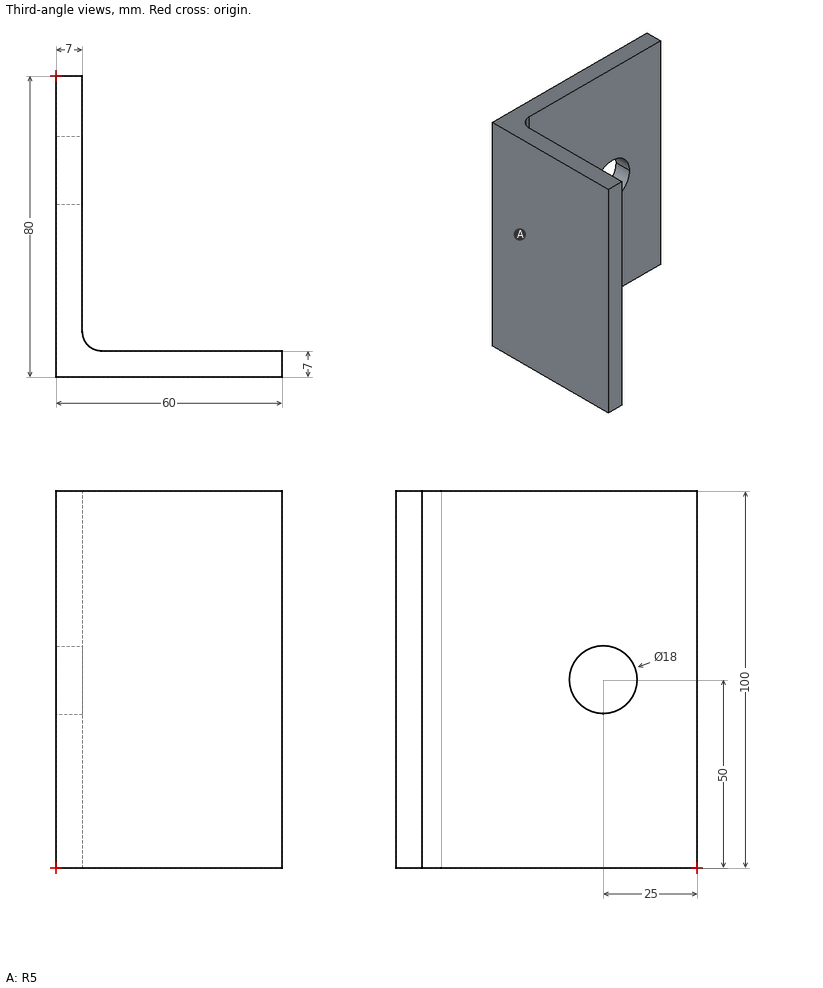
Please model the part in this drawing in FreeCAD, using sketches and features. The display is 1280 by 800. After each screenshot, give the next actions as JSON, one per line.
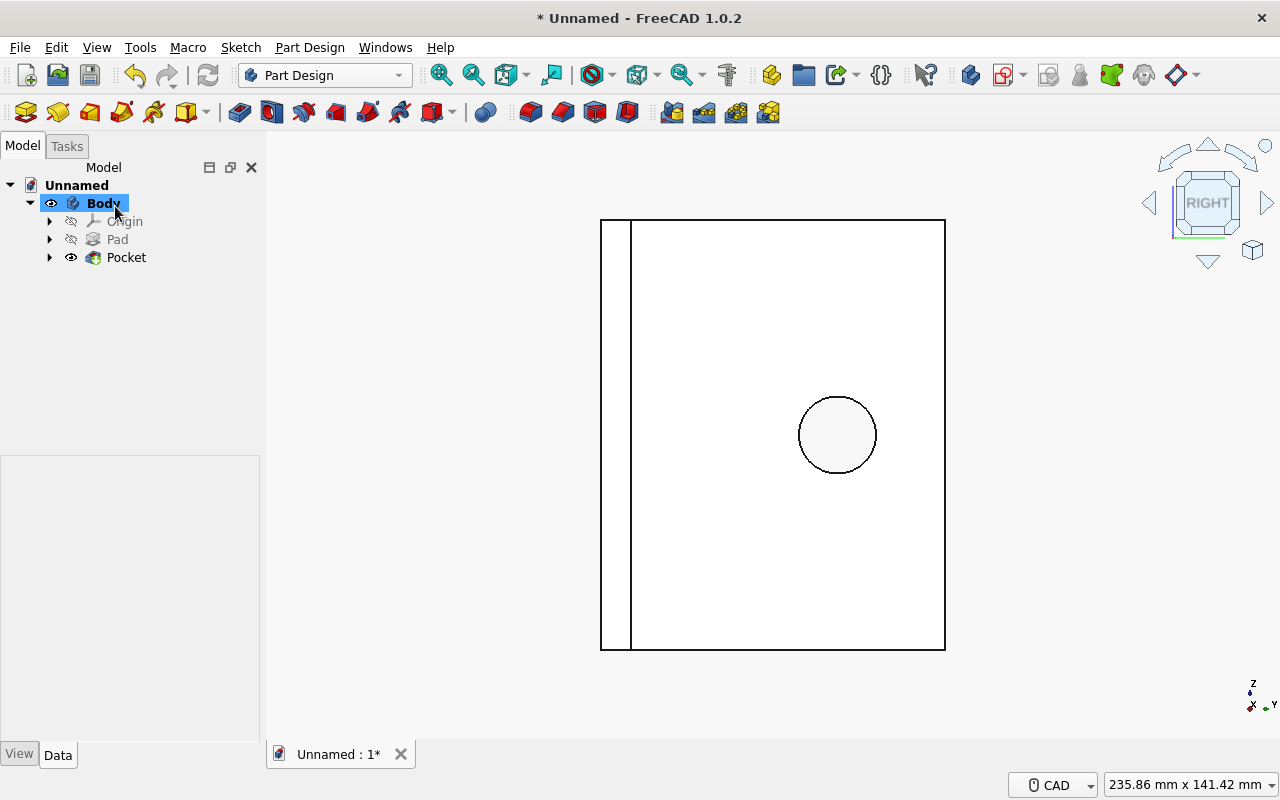
{"action": "key", "text": "5"}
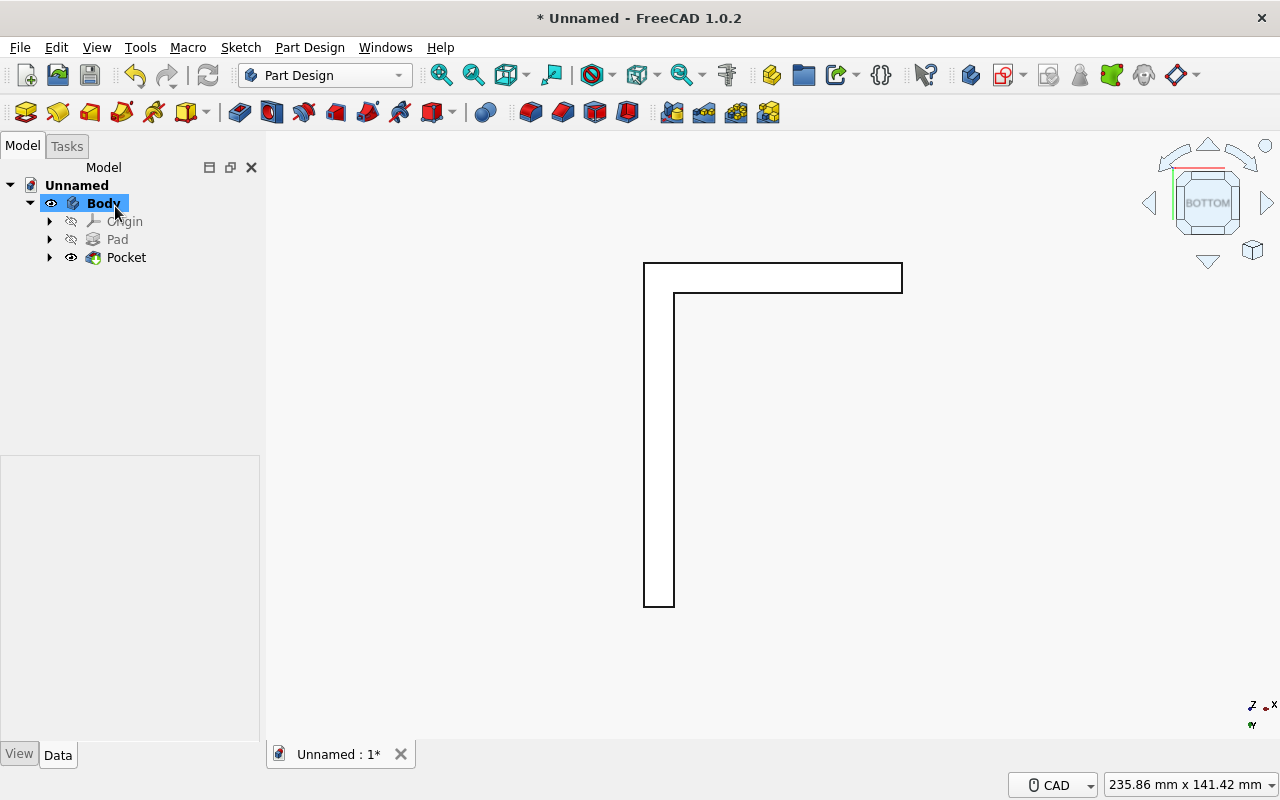
{"action": "key", "text": "4"}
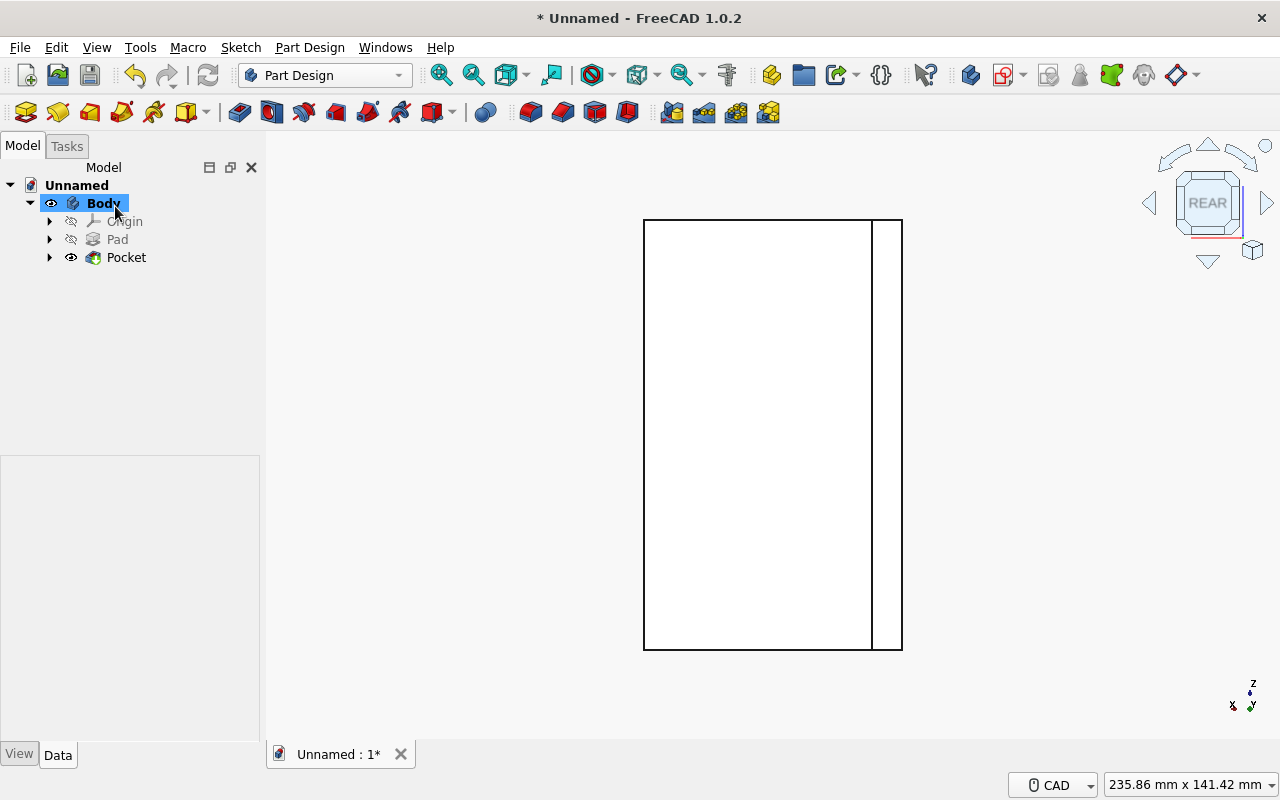
{"action": "key", "text": "6"}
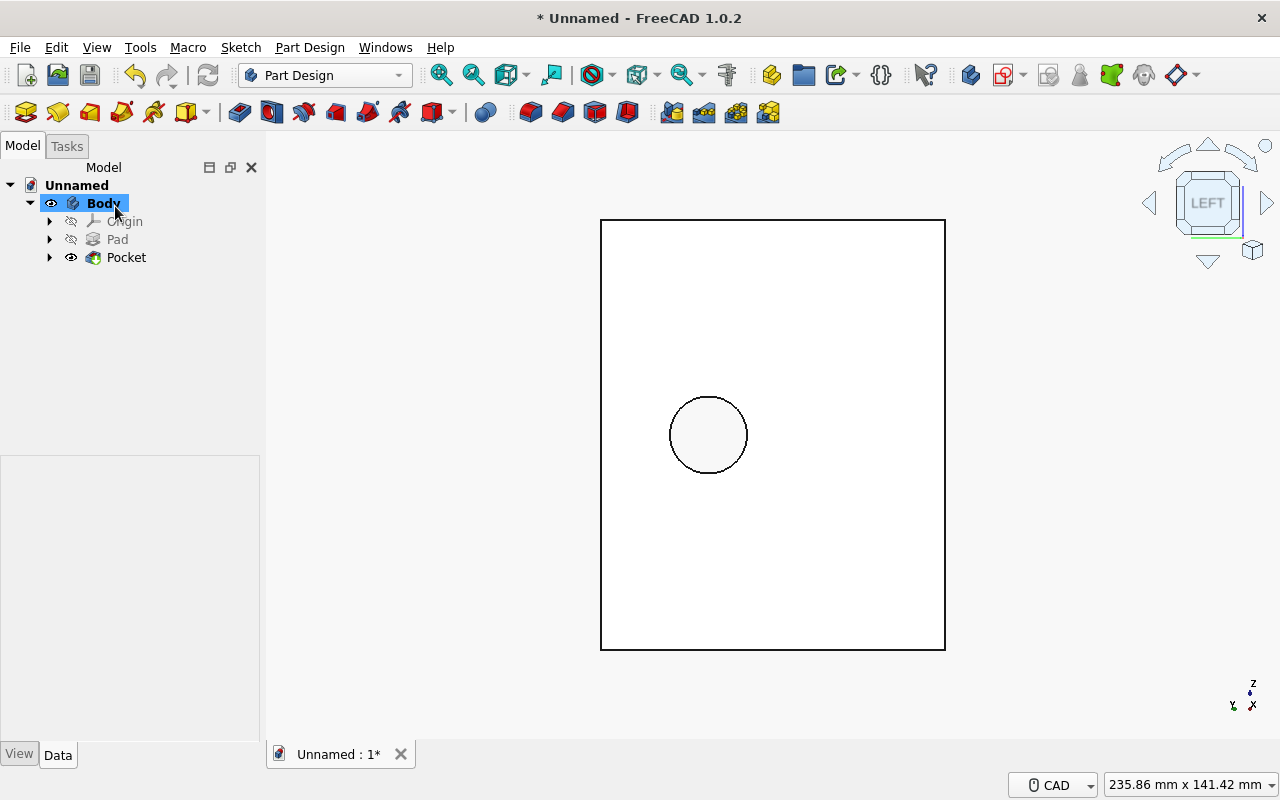
{"action": "key", "text": "v 3"}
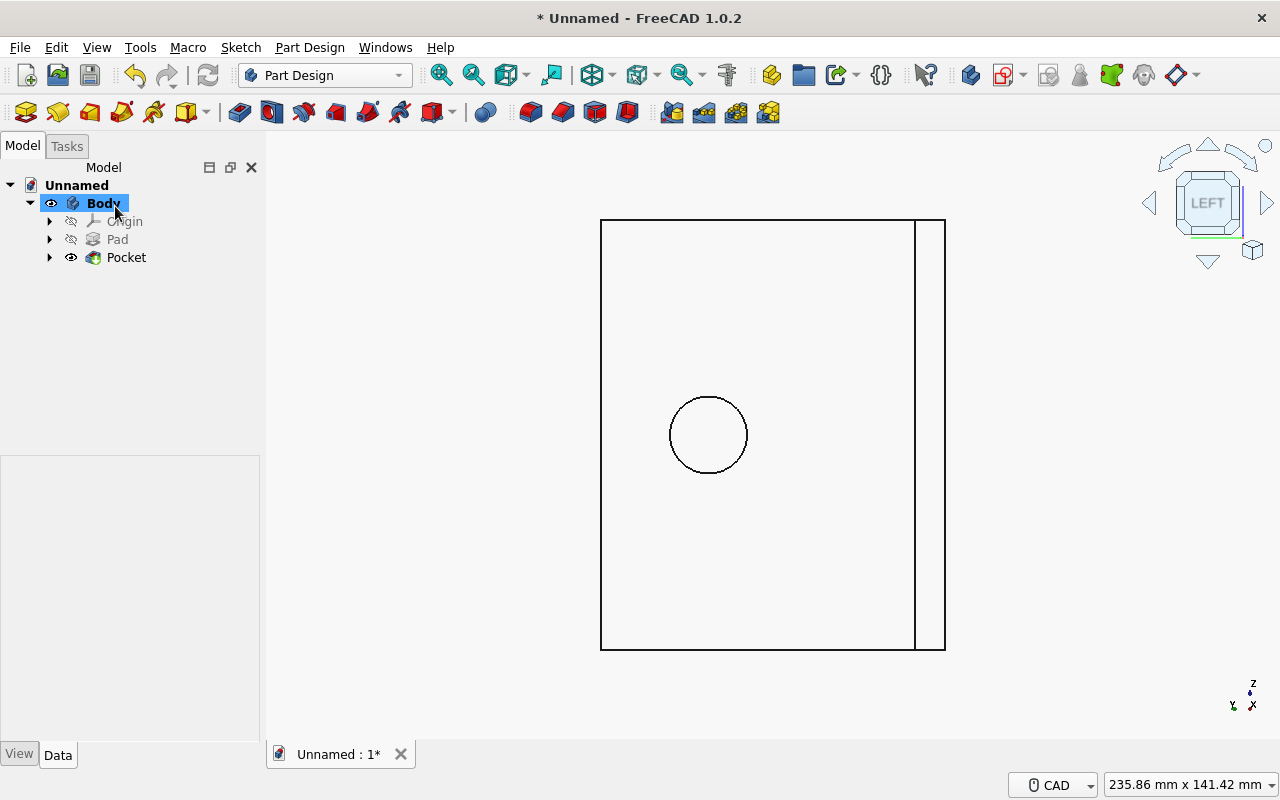
{"action": "key", "text": "0"}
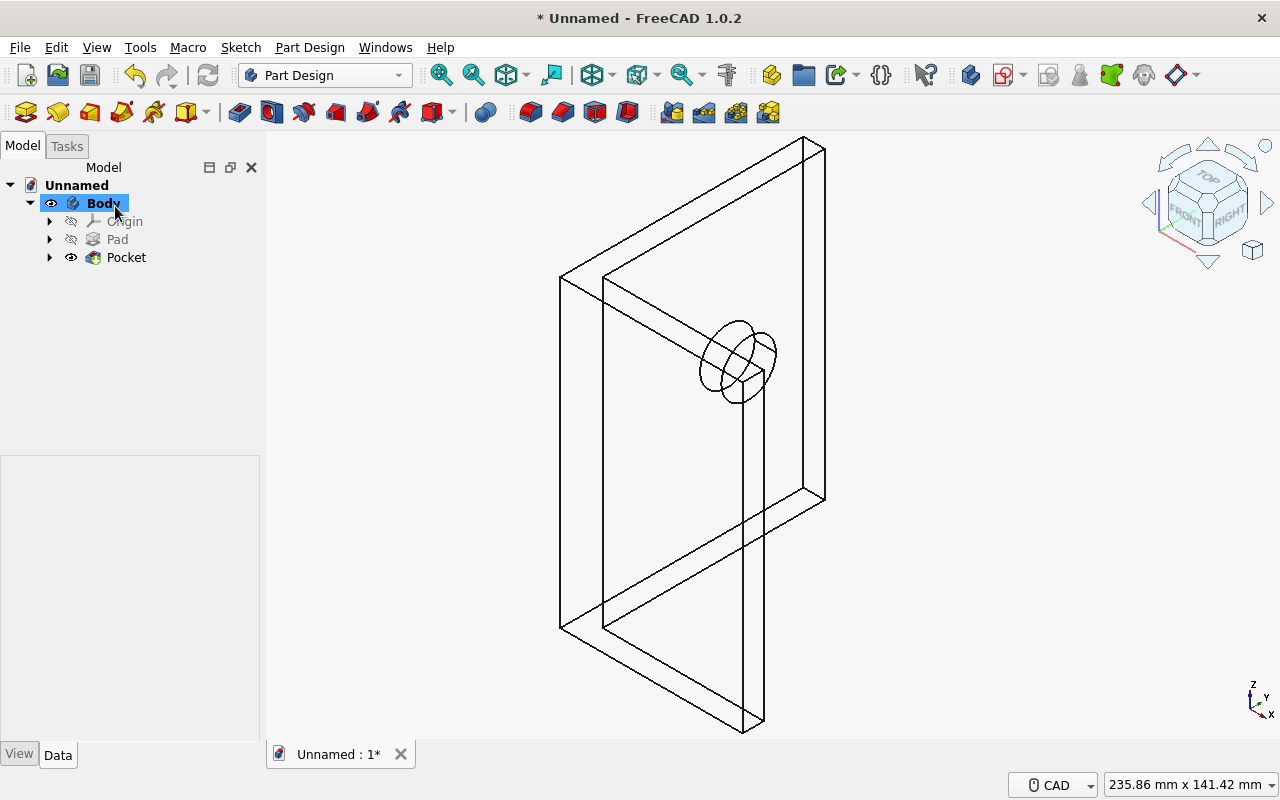
{"action": "left_click", "coordinate": [603, 452]}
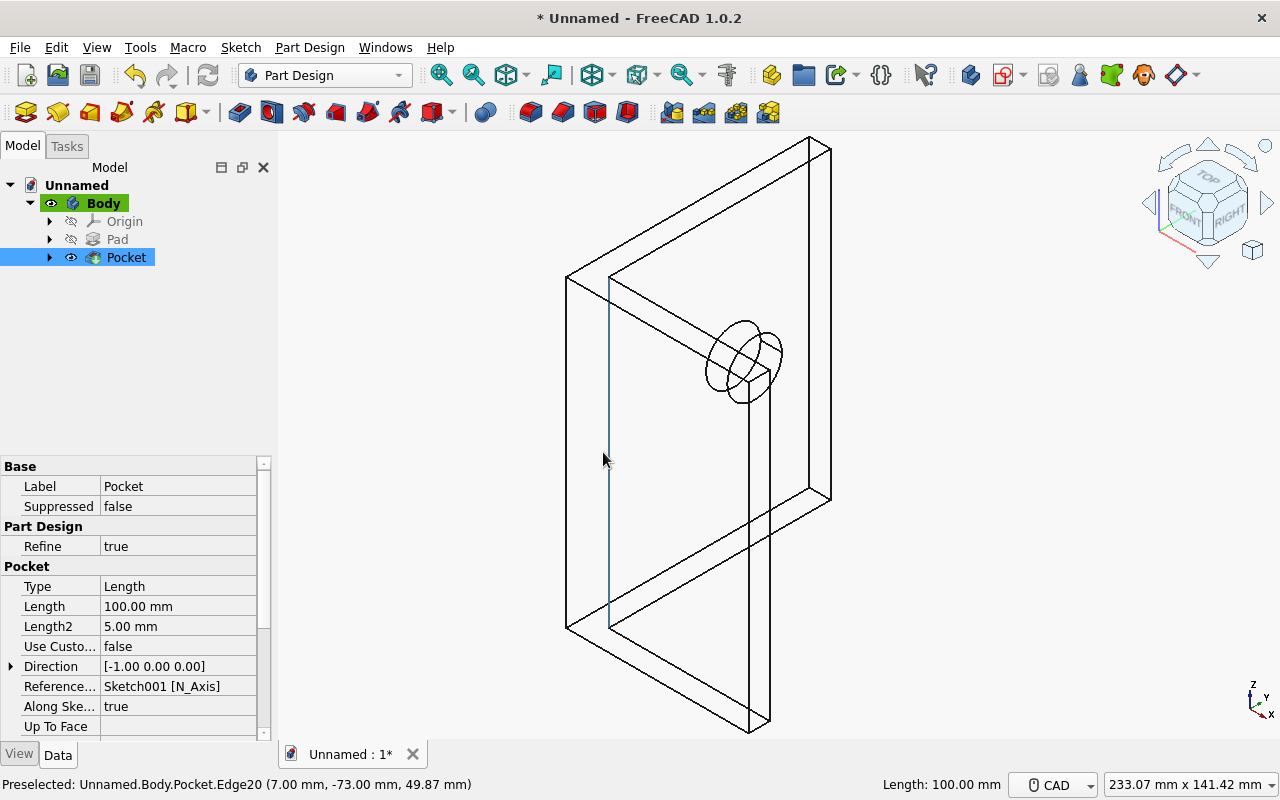
{"action": "key", "text": "v 1"}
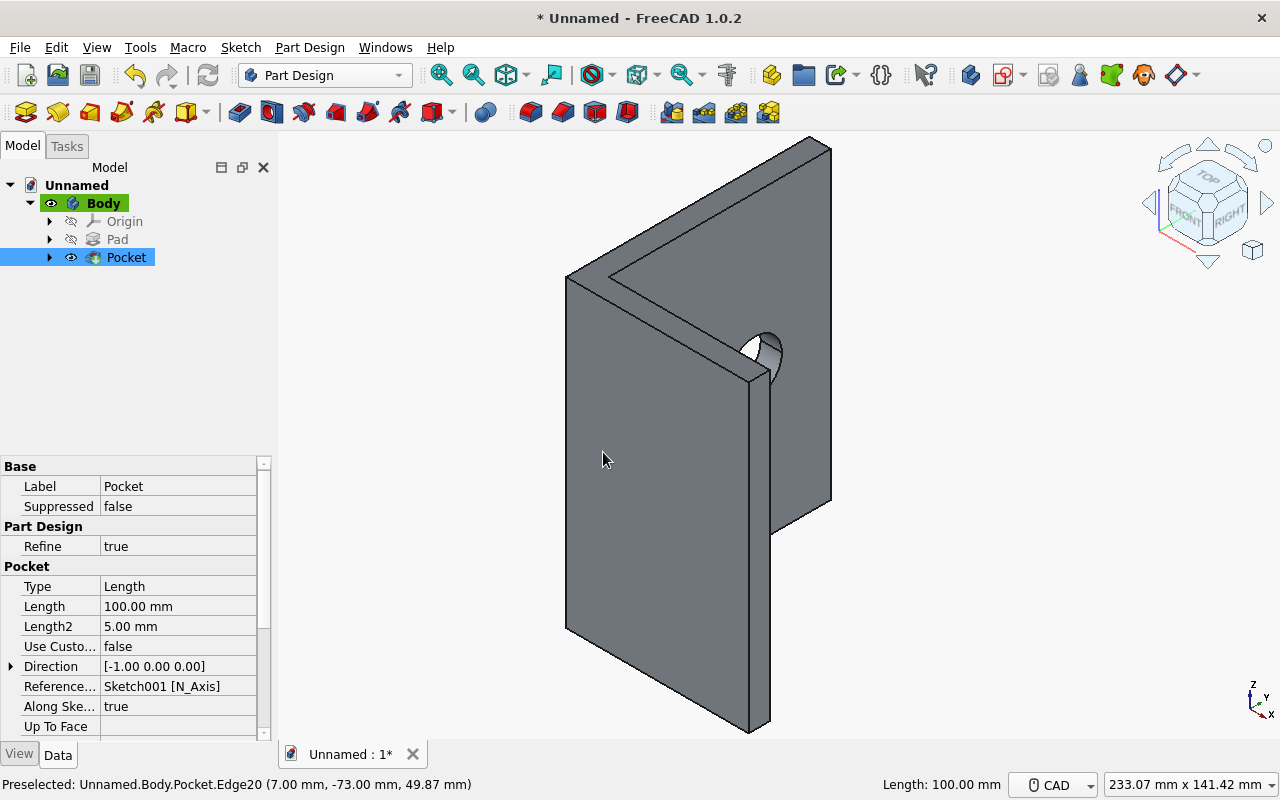
{"action": "left_click", "coordinate": [532, 112]}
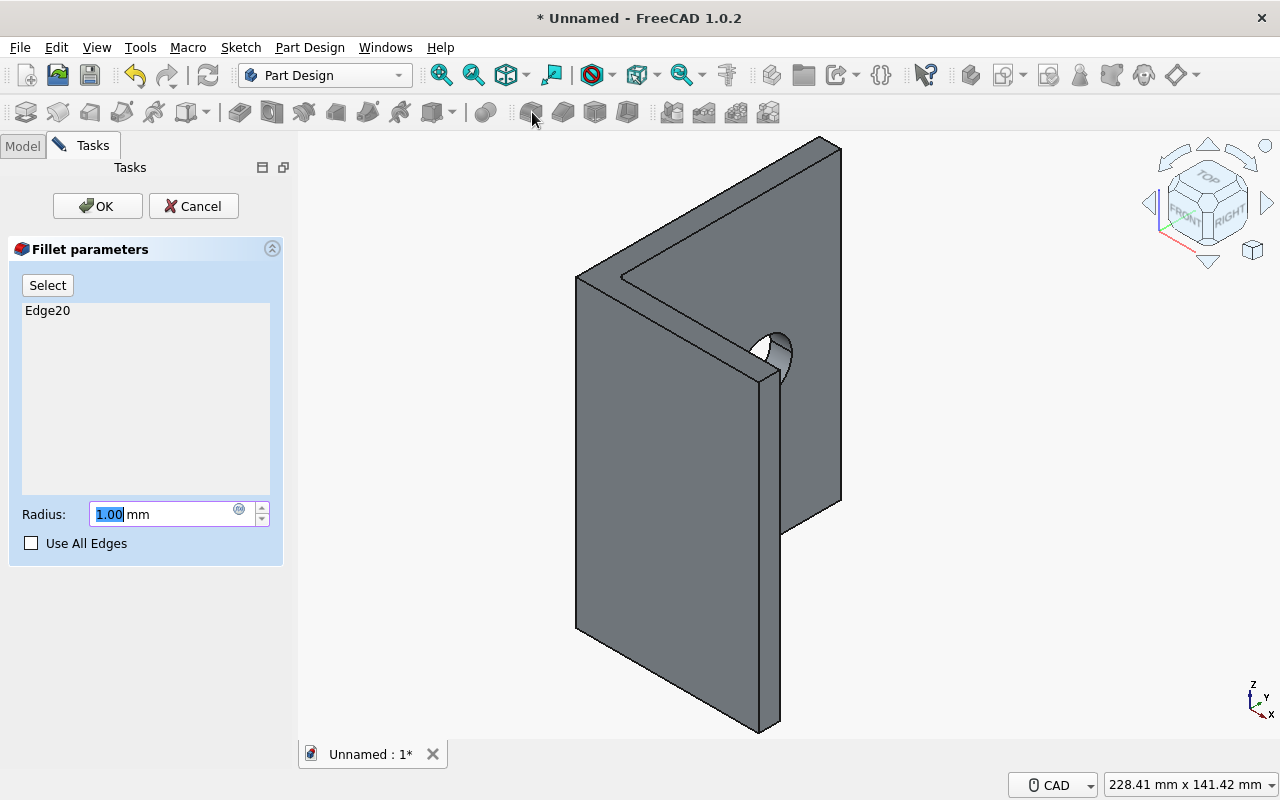
{"action": "type", "text": "5"}
{"action": "key", "text": "Tab"}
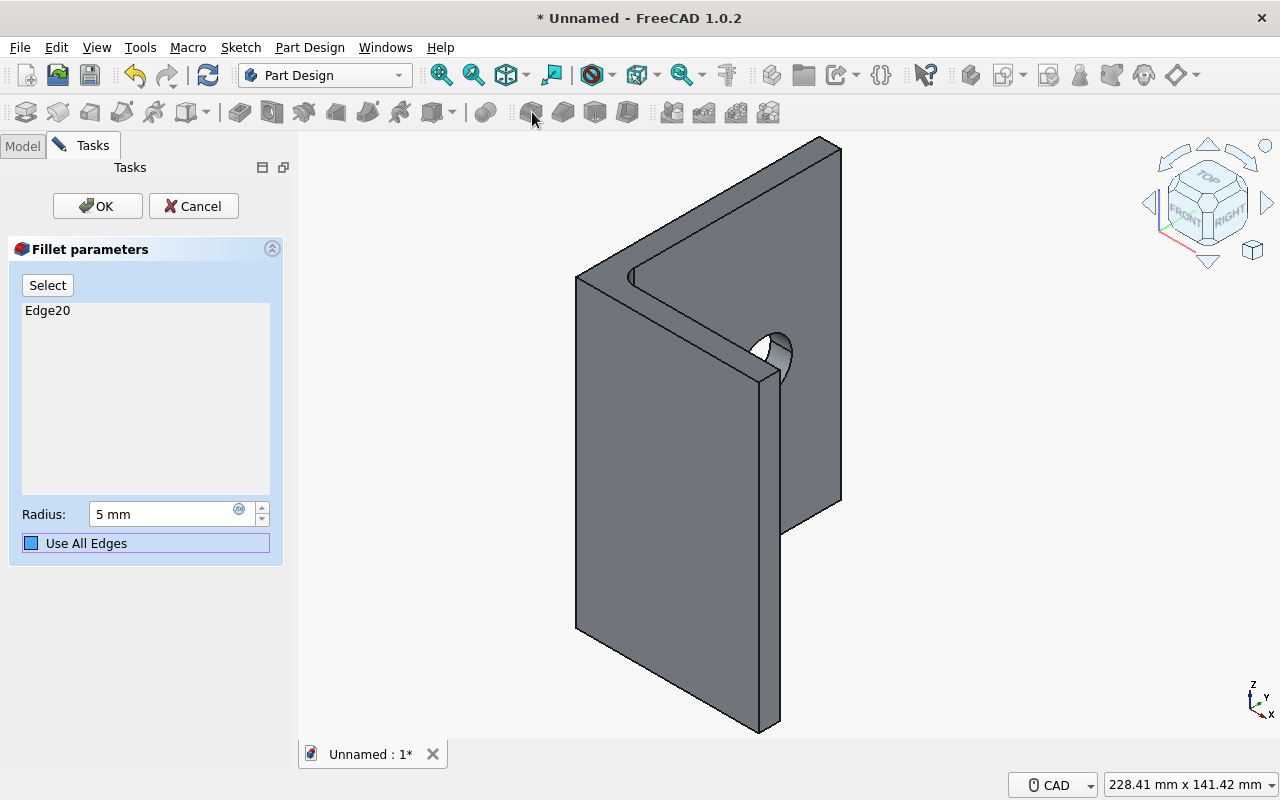
{"action": "left_click", "coordinate": [98, 206]}